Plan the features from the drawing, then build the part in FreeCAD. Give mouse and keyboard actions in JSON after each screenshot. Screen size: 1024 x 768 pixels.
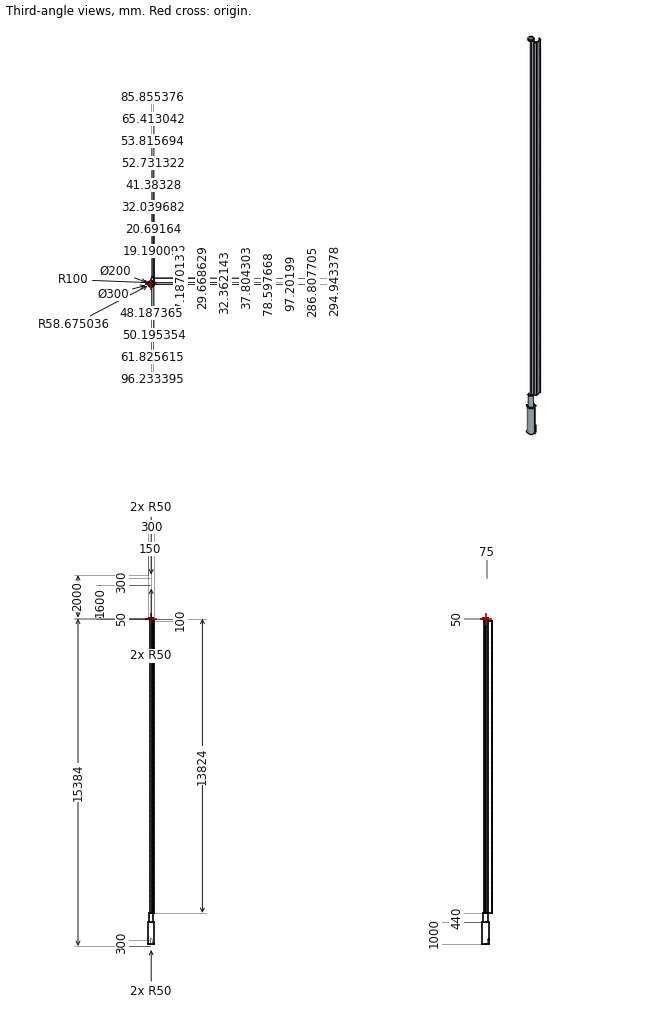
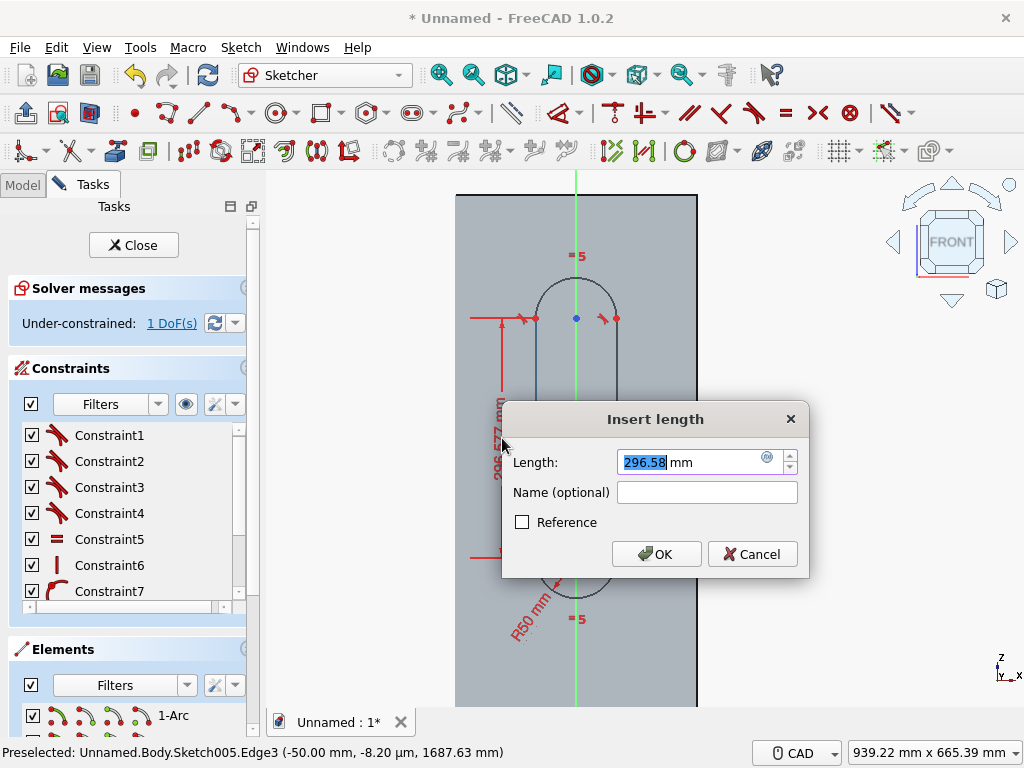
{"action": "type", "text": "300"}
{"action": "key", "text": "Return"}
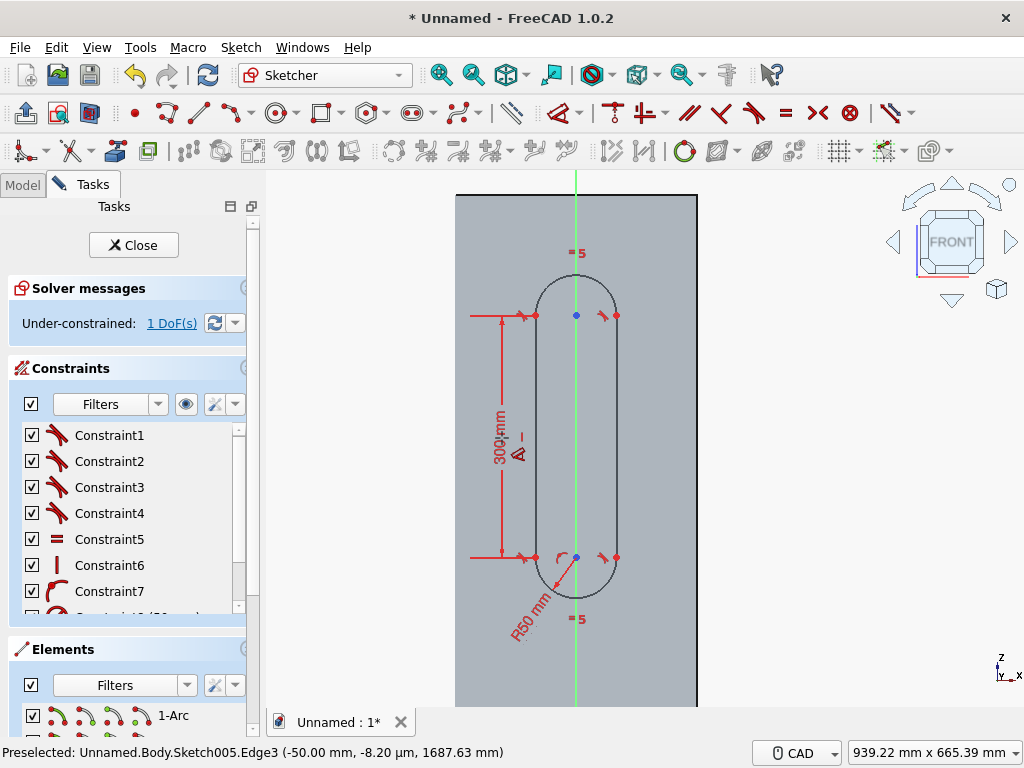
{"action": "left_click", "coordinate": [536, 558]}
{"action": "left_click", "coordinate": [502, 590]}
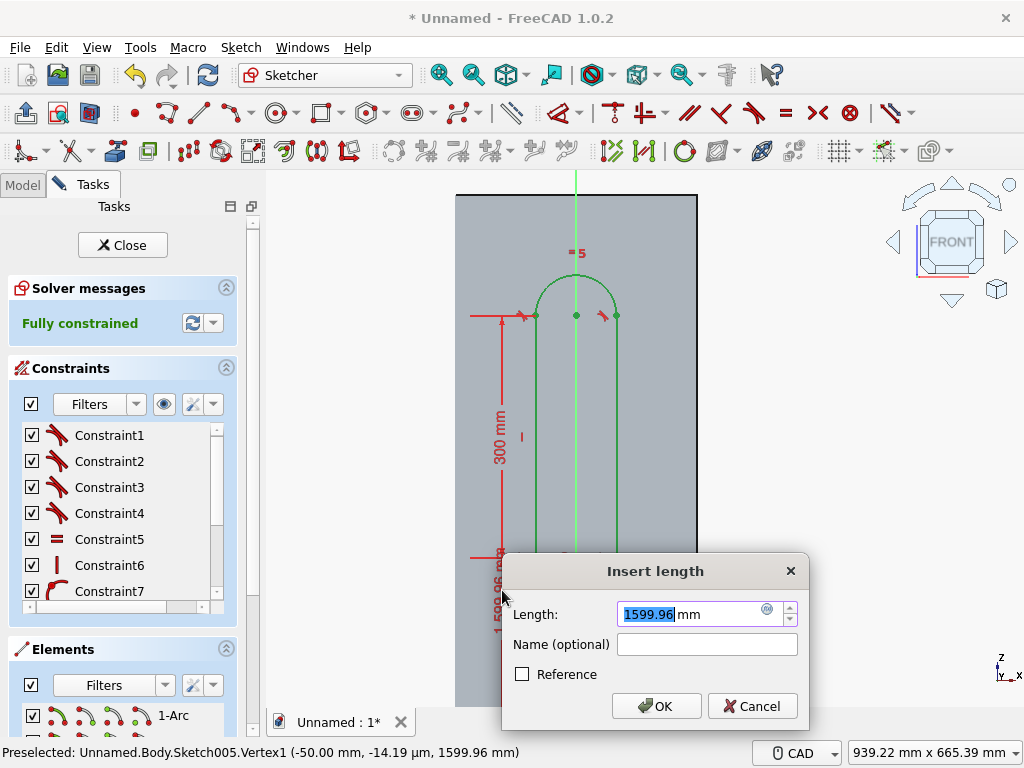
{"action": "type", "text": "1600"}
{"action": "key", "text": "Return"}
{"action": "key", "text": "Escape"}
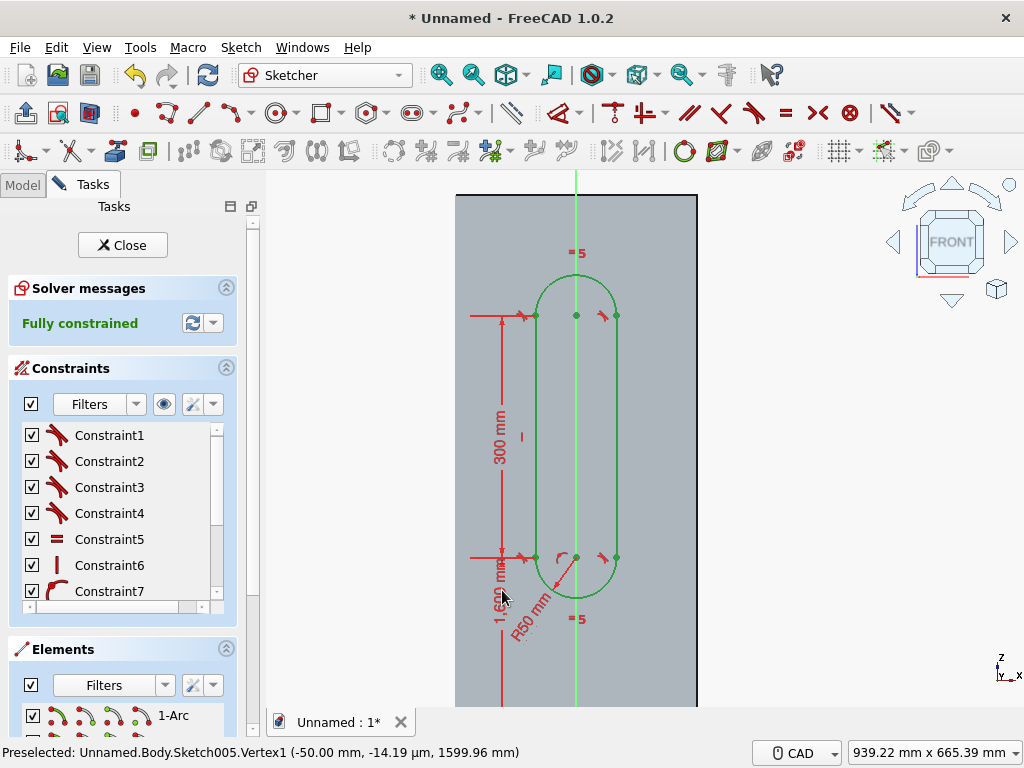
{"action": "left_click", "coordinate": [123, 245]}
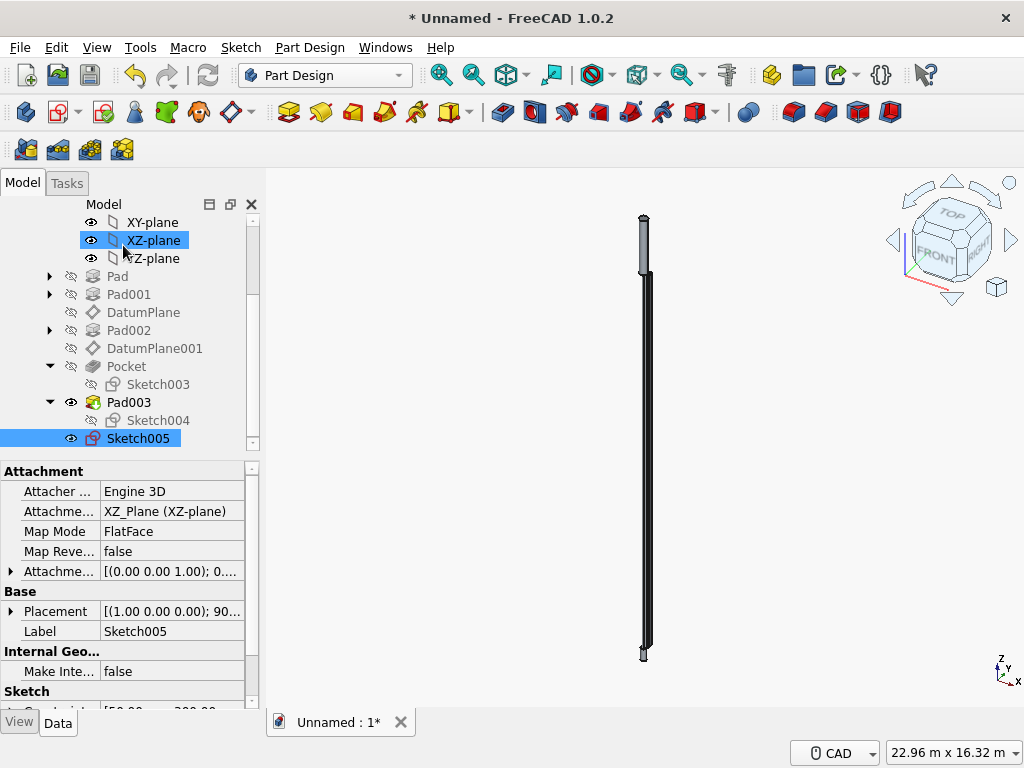
{"action": "left_click", "coordinate": [504, 112]}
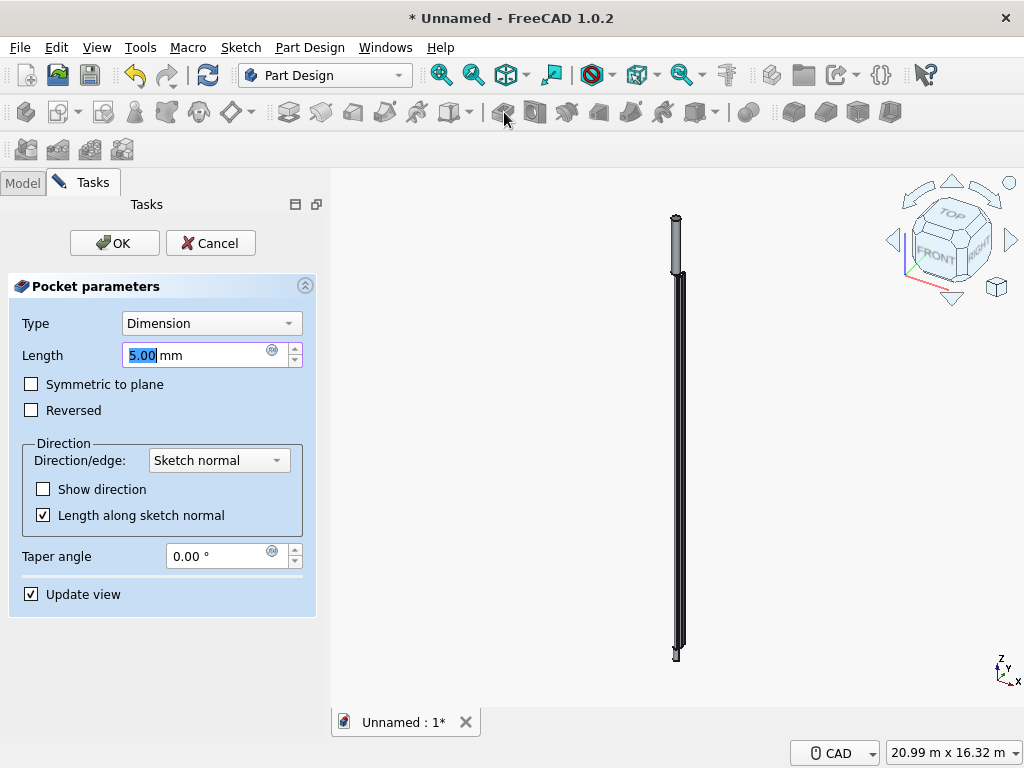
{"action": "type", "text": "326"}
{"action": "key", "text": "Tab"}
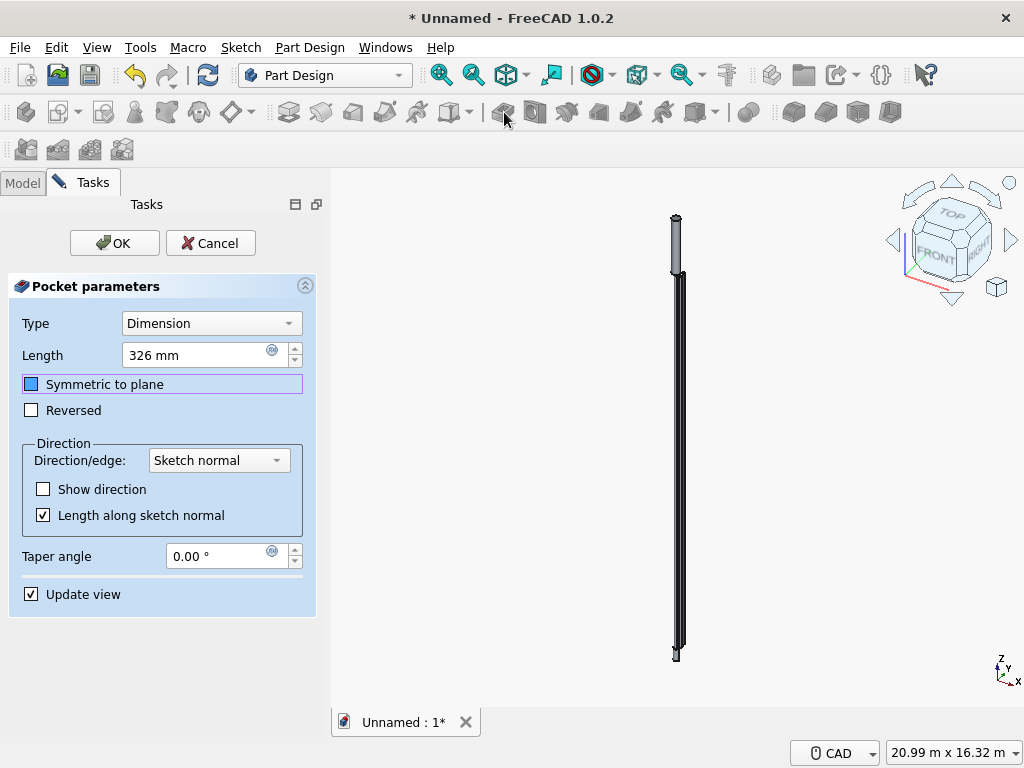
{"action": "left_click", "coordinate": [115, 243]}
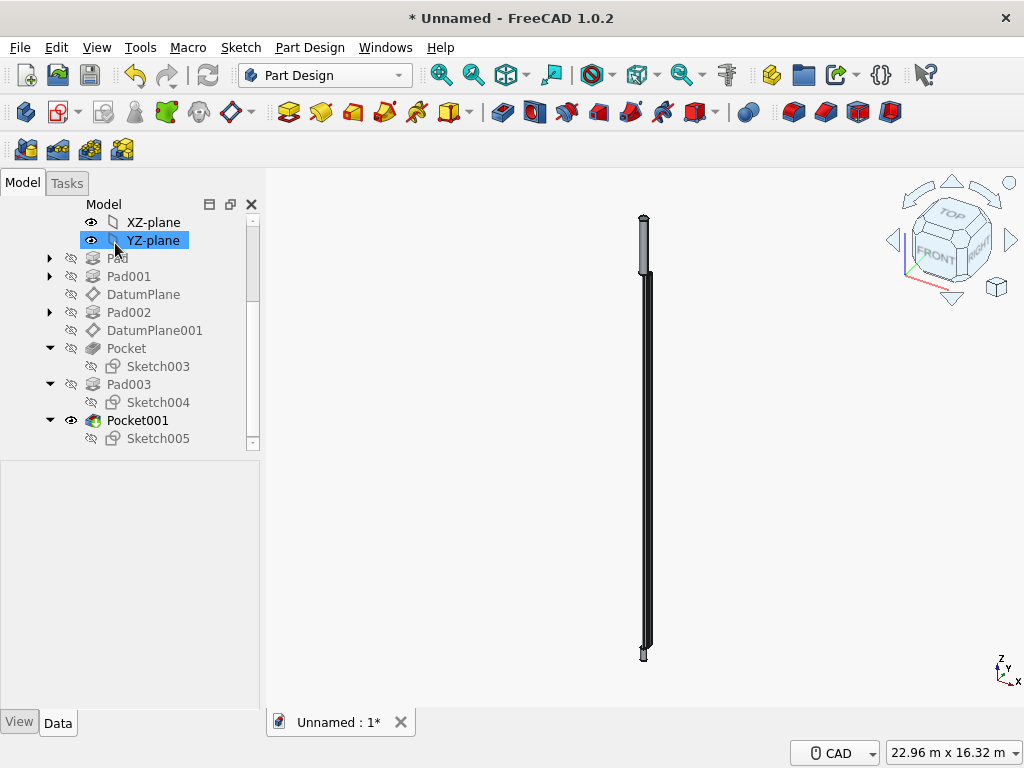
{"action": "left_click", "coordinate": [58, 112]}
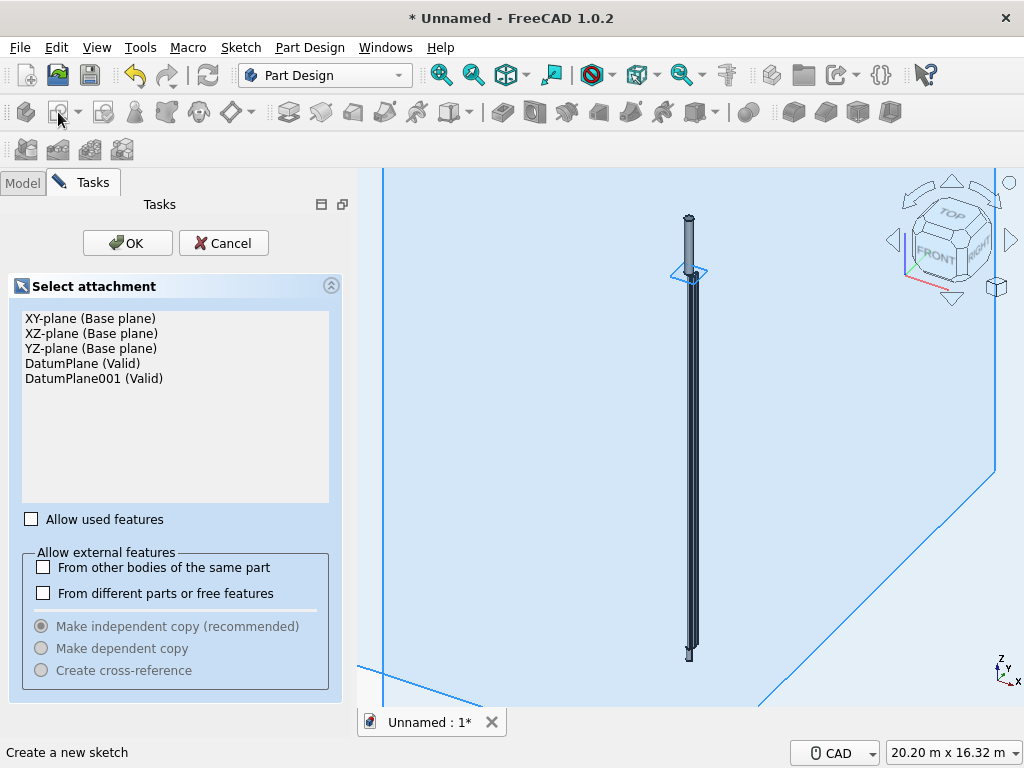
{"action": "left_click", "coordinate": [82, 334]}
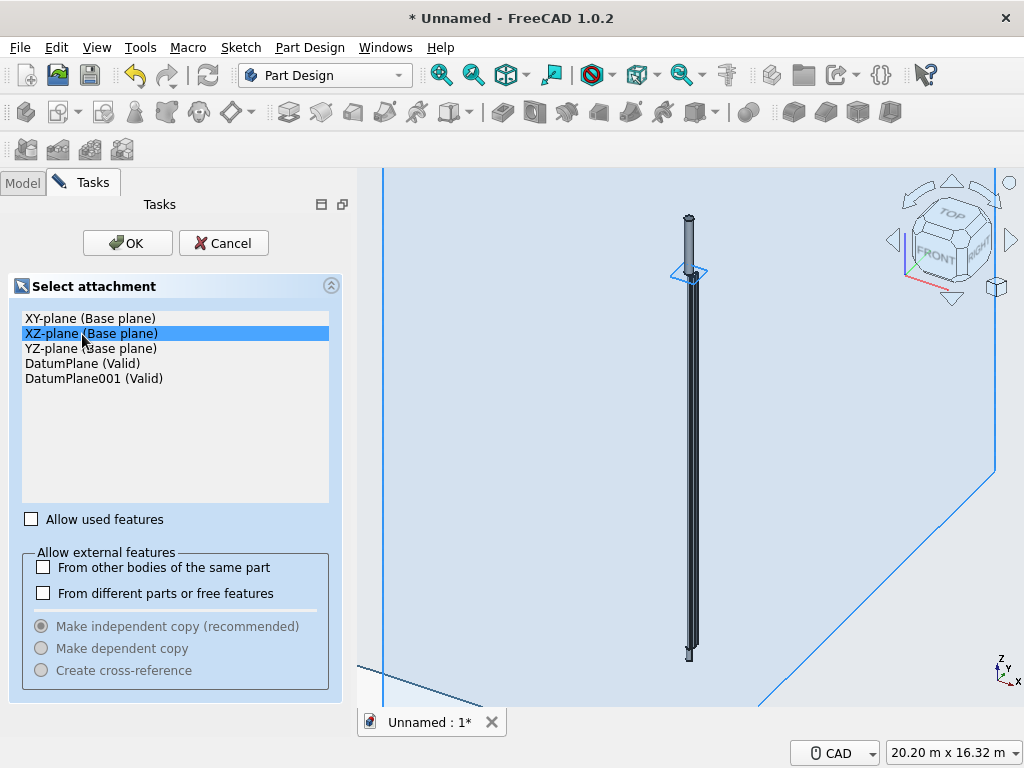
{"action": "left_click", "coordinate": [128, 243]}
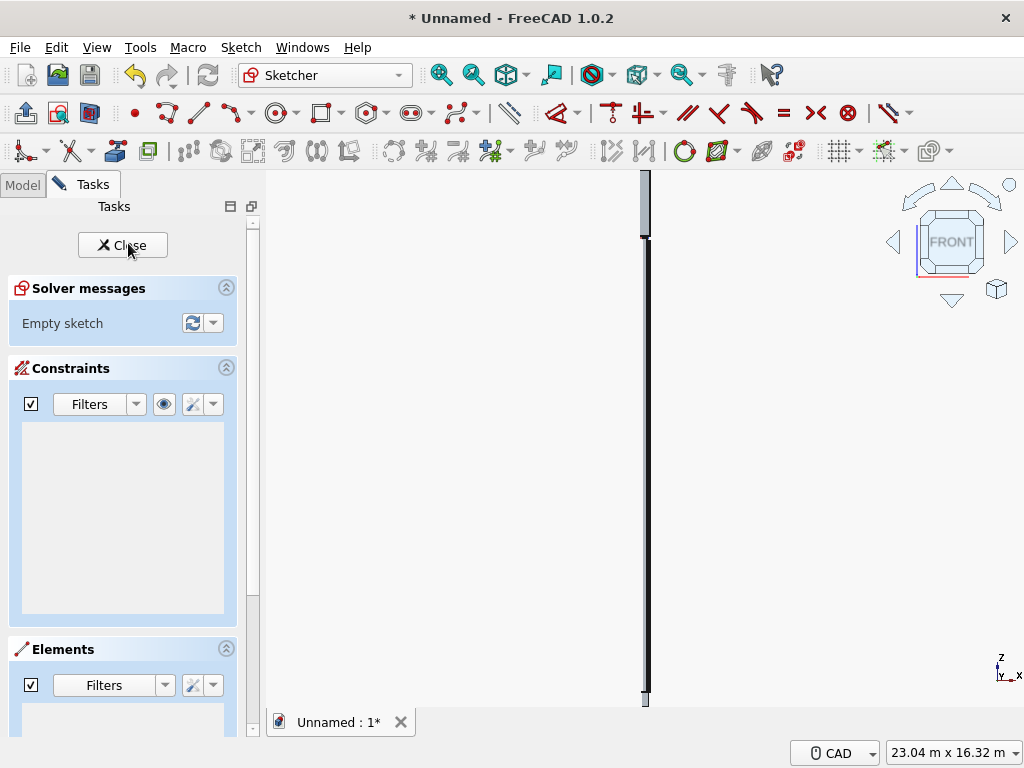
{"action": "left_click", "coordinate": [90, 114]}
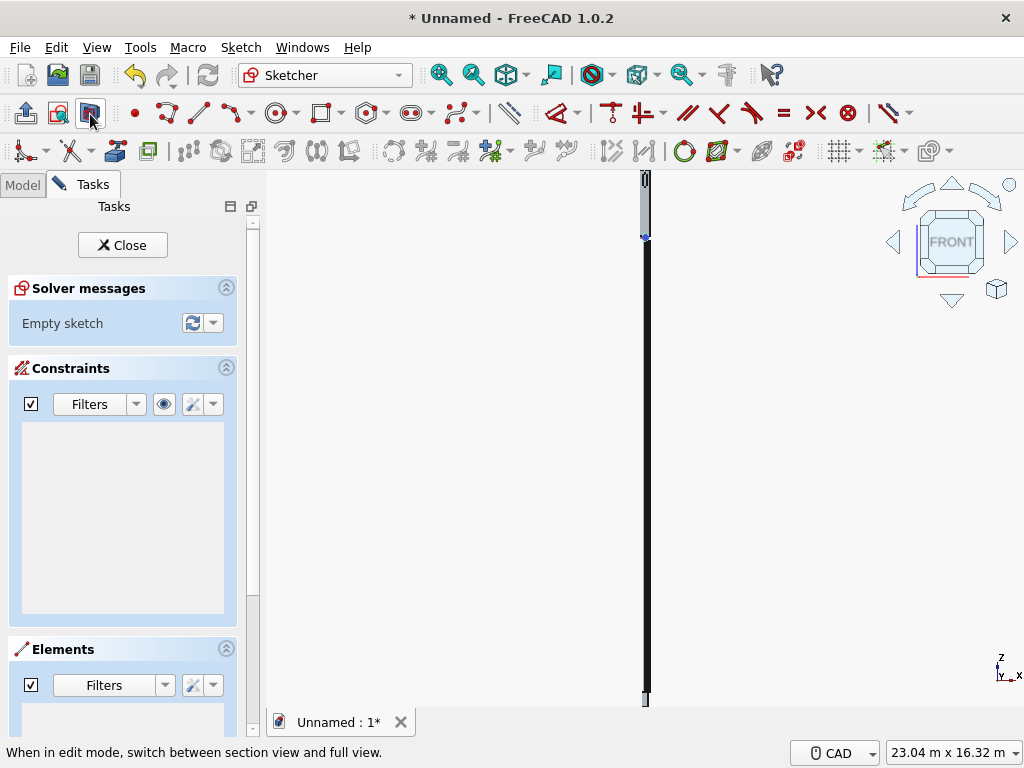
{"action": "scroll", "coordinate": [576, 438], "scroll_direction": "down", "scroll_amount": 5}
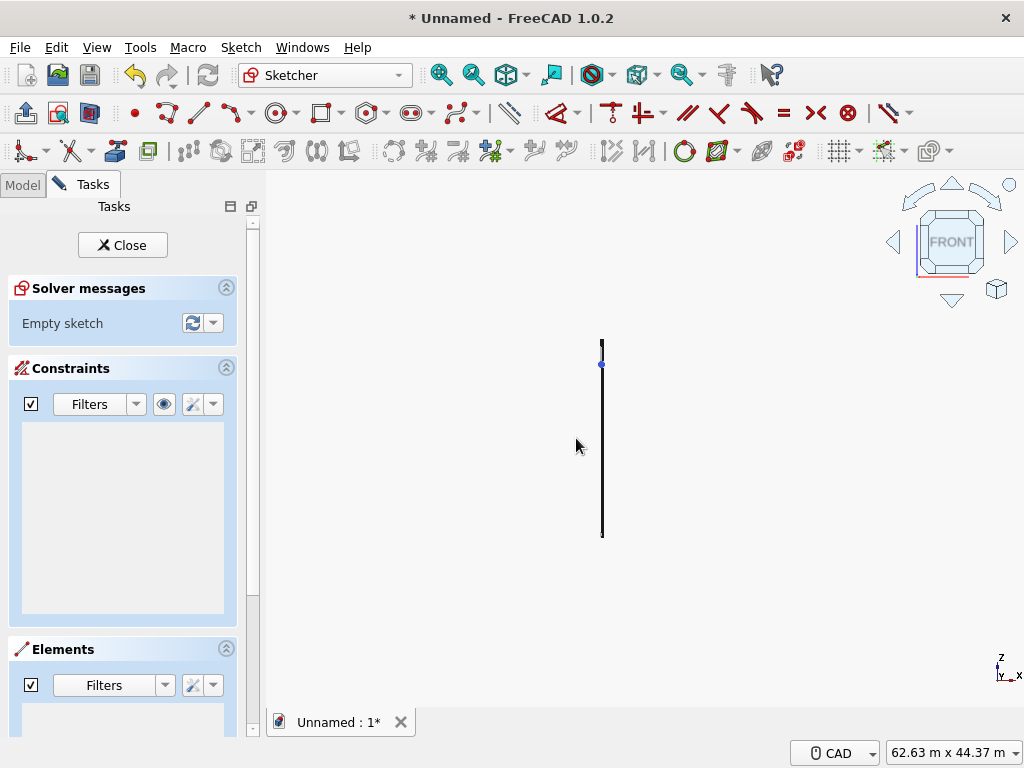
{"action": "scroll", "coordinate": [603, 338], "scroll_direction": "up", "scroll_amount": 15}